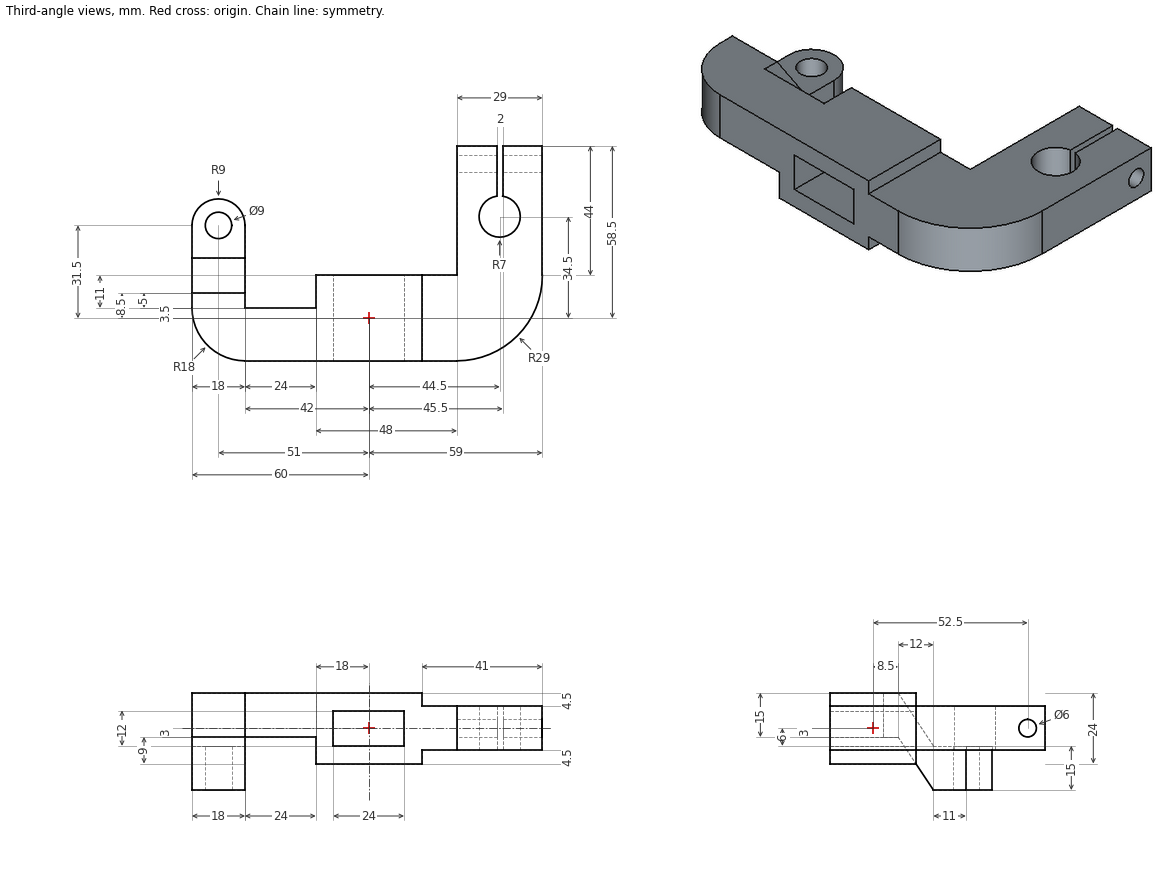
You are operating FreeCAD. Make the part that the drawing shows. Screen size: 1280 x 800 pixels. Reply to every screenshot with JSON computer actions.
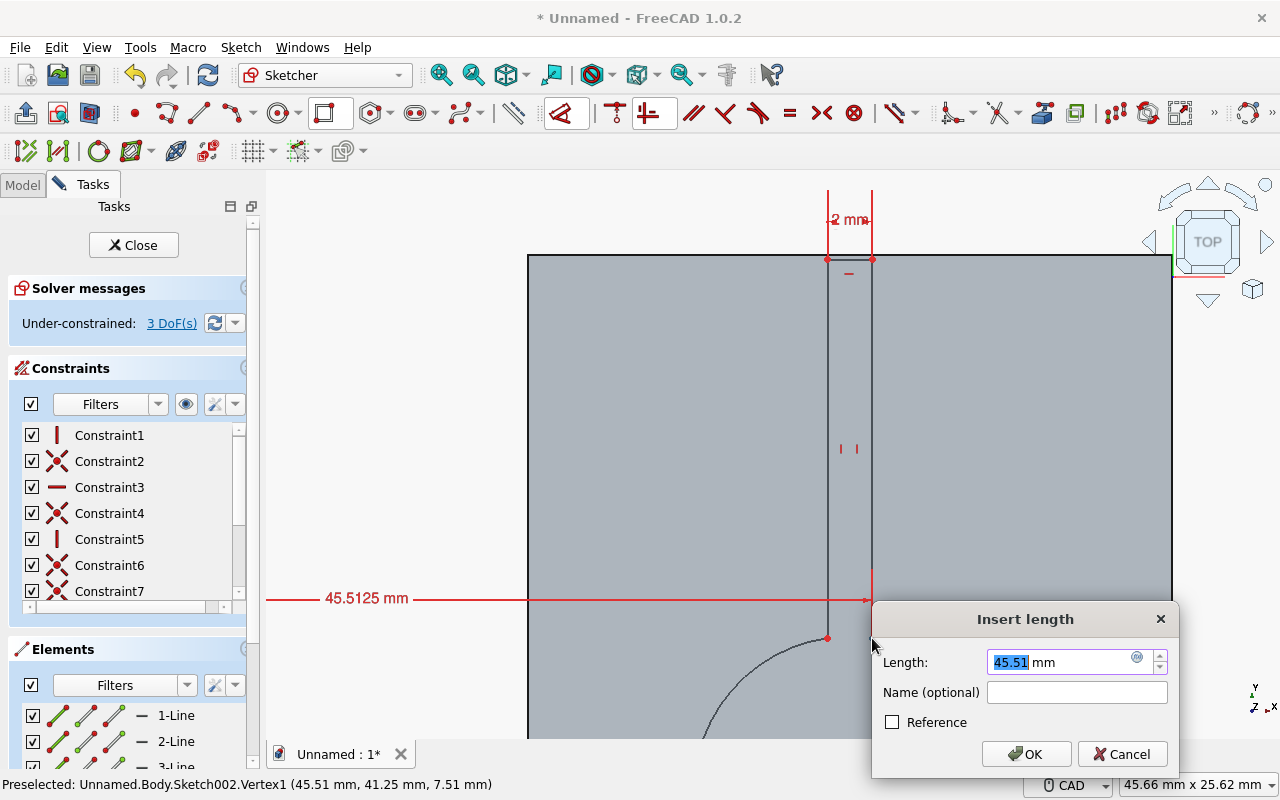
{"action": "type", "text": "45.5"}
{"action": "key", "text": "Return"}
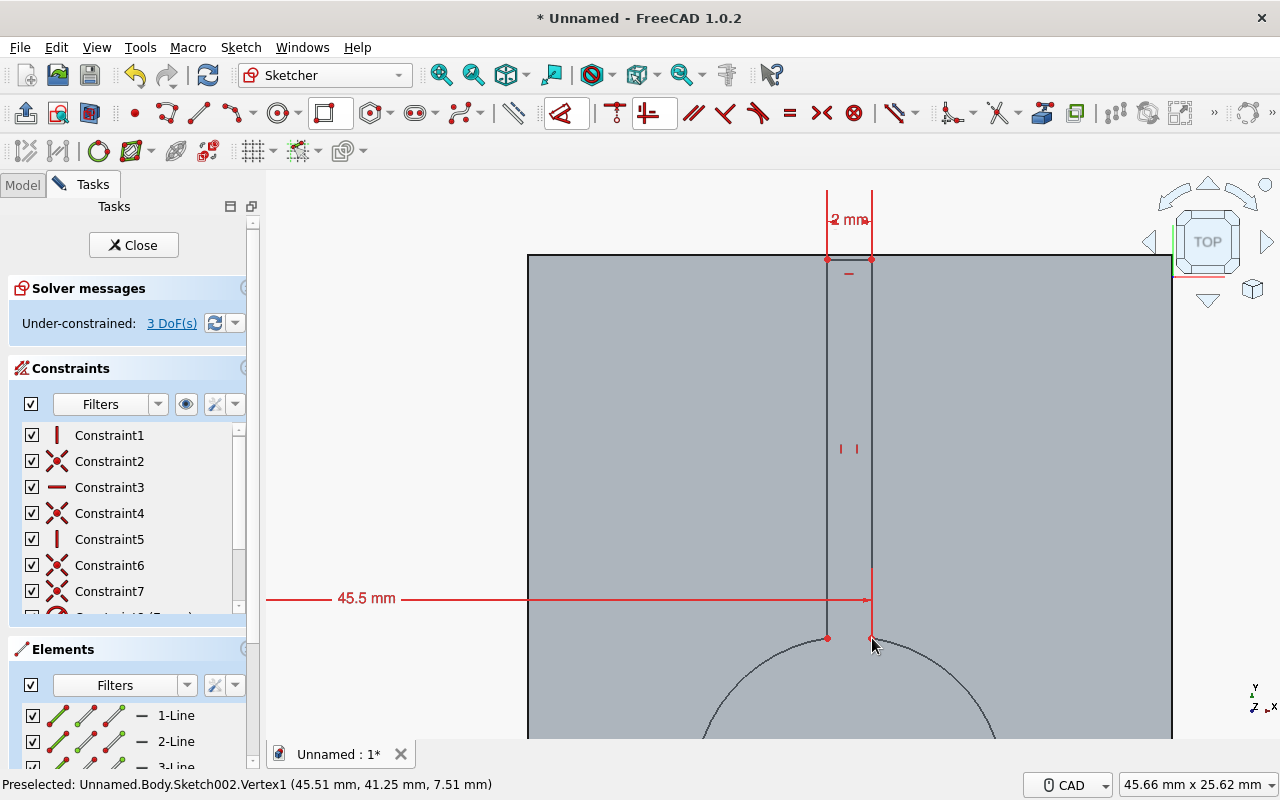
{"action": "left_click", "coordinate": [872, 260]}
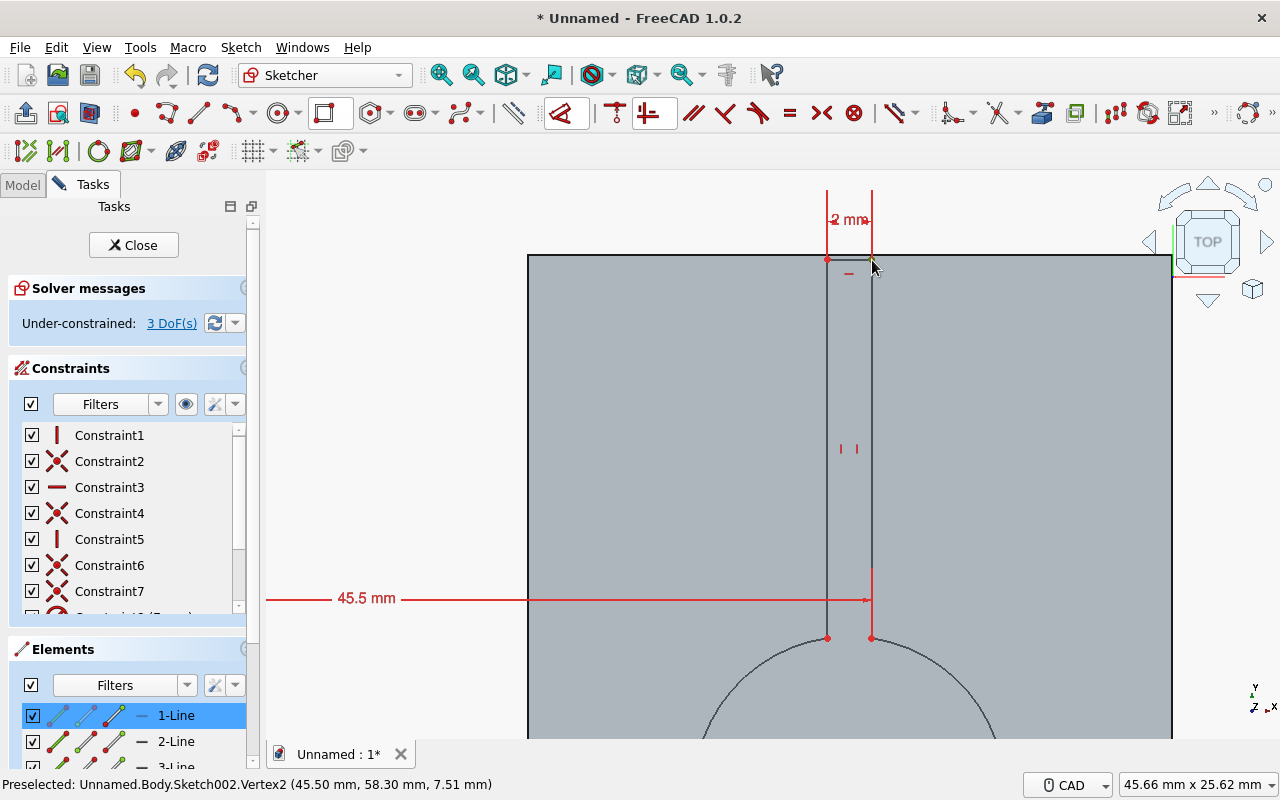
{"action": "left_click", "coordinate": [584, 114]}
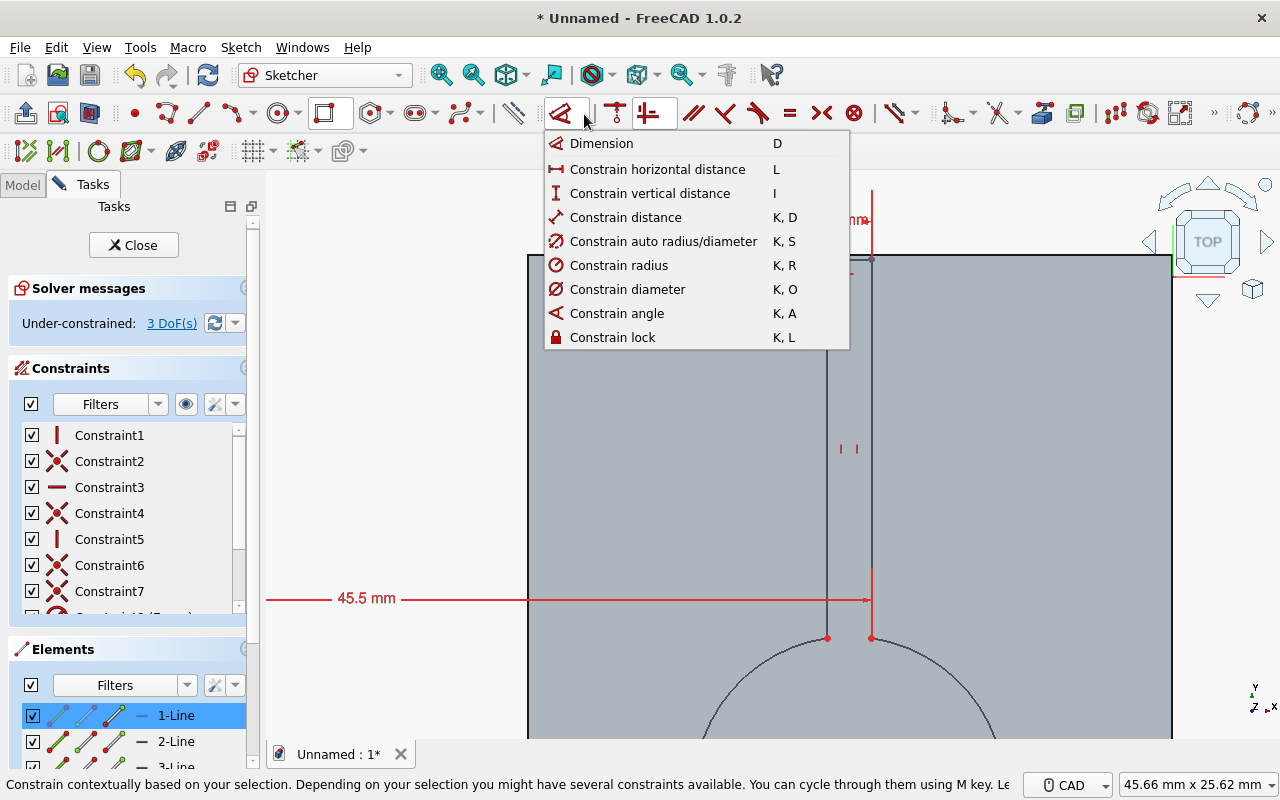
{"action": "left_click", "coordinate": [697, 193]}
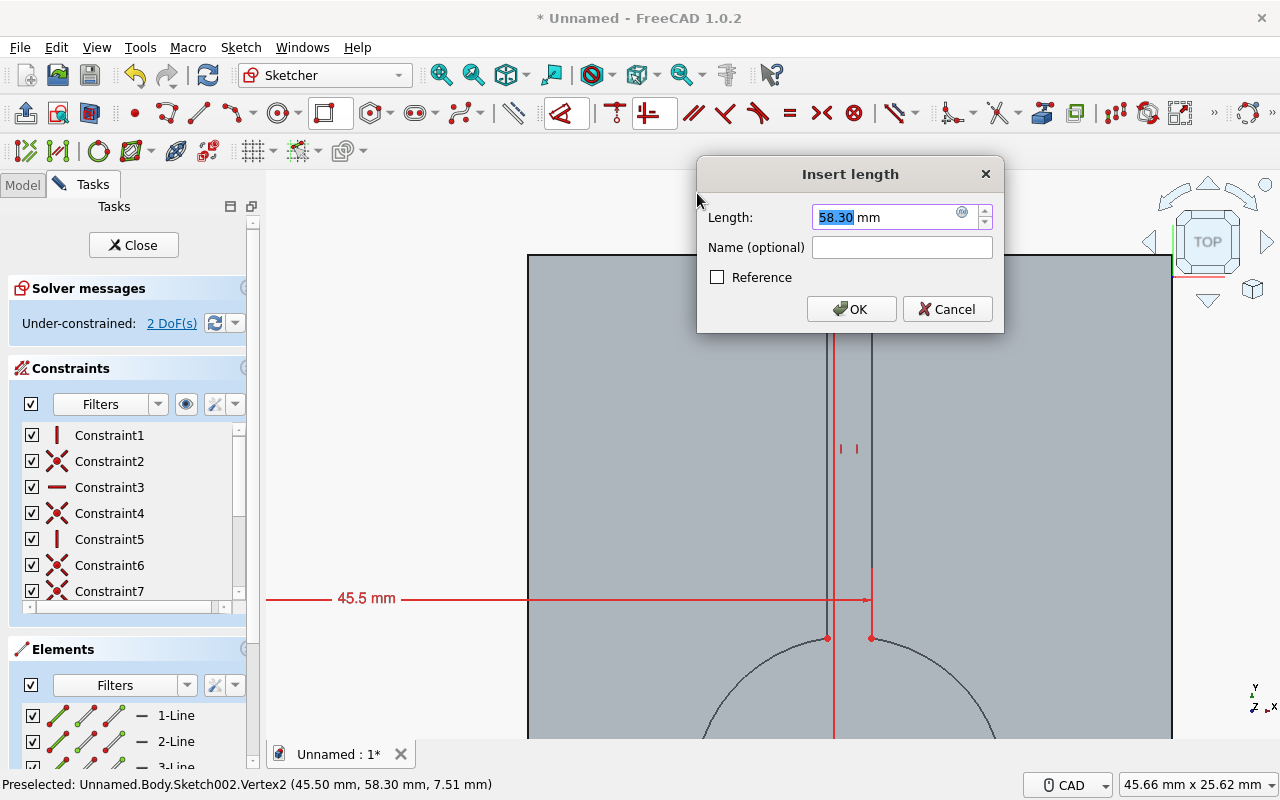
{"action": "type", "text": "58.5"}
{"action": "key", "text": "Return"}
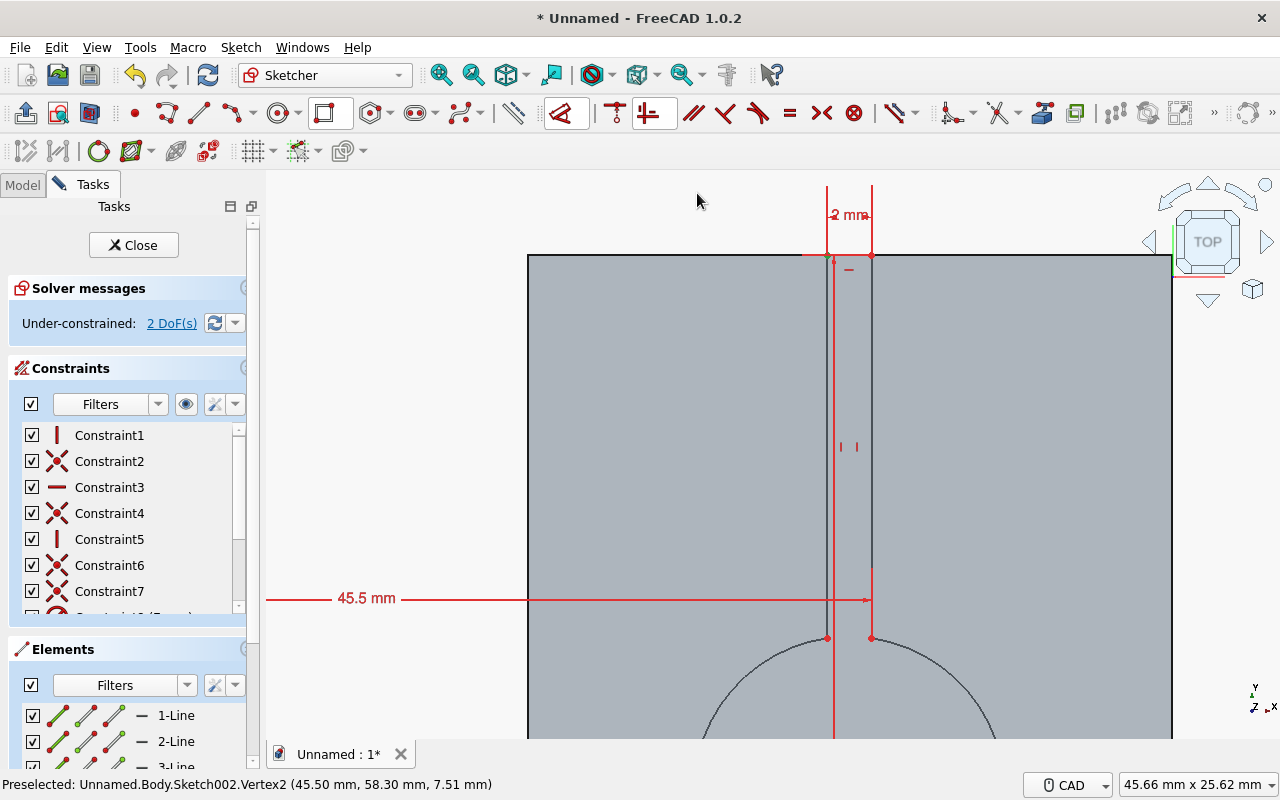
{"action": "scroll", "coordinate": [850, 260], "scroll_direction": "down", "scroll_amount": 6}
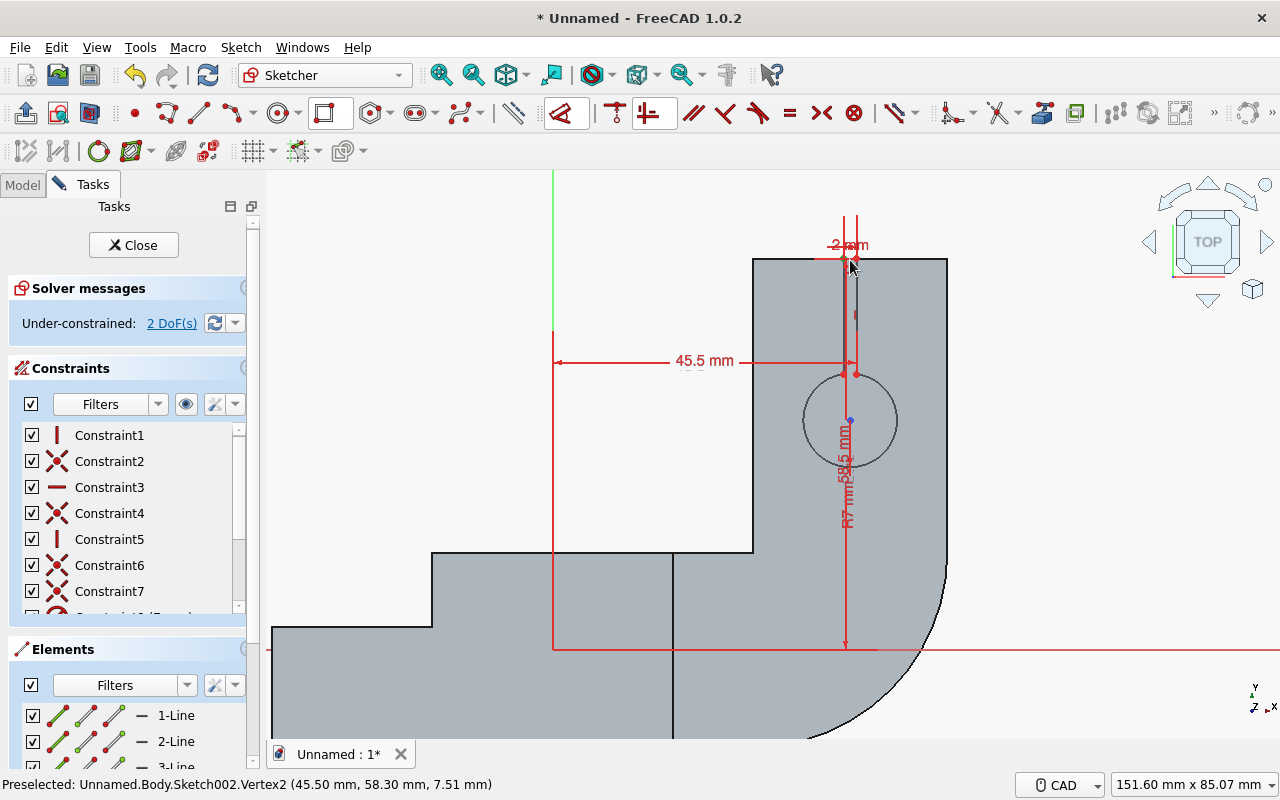
{"action": "left_click", "coordinate": [850, 420]}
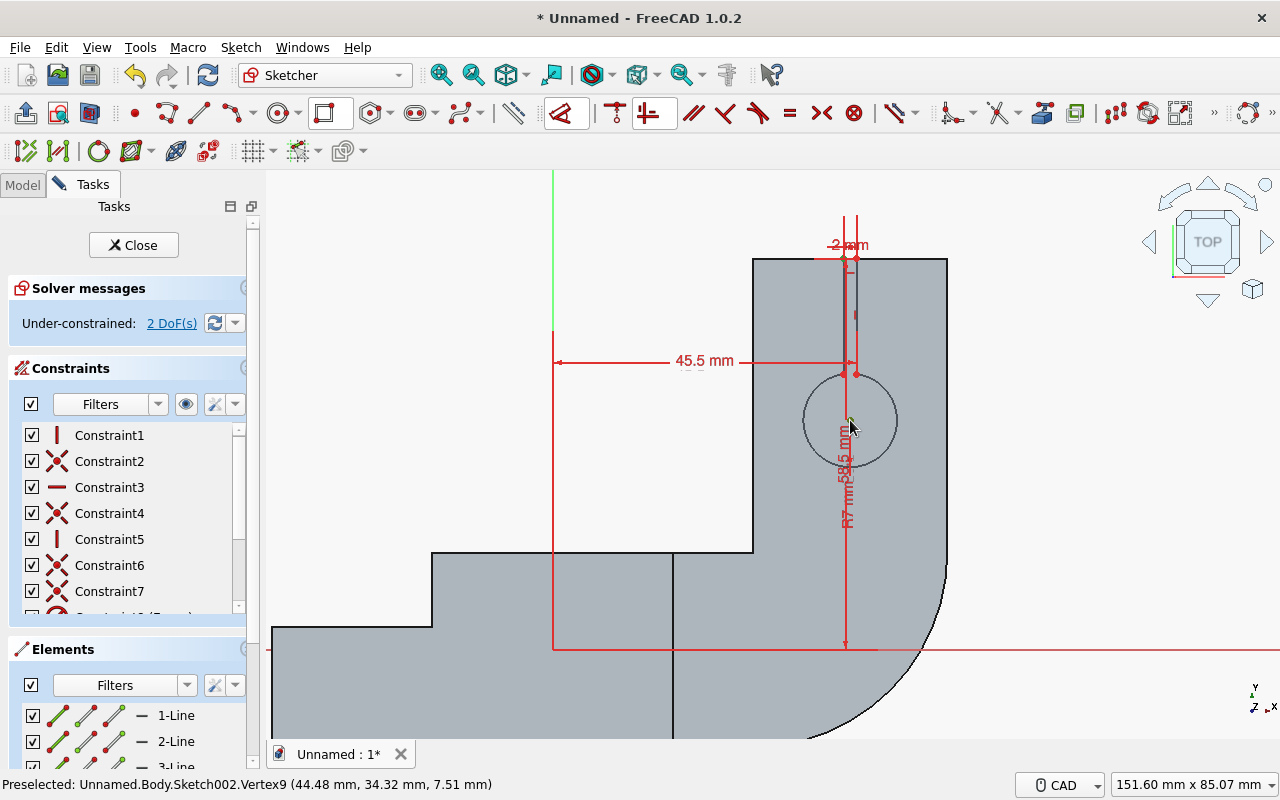
{"action": "key", "text": "l"}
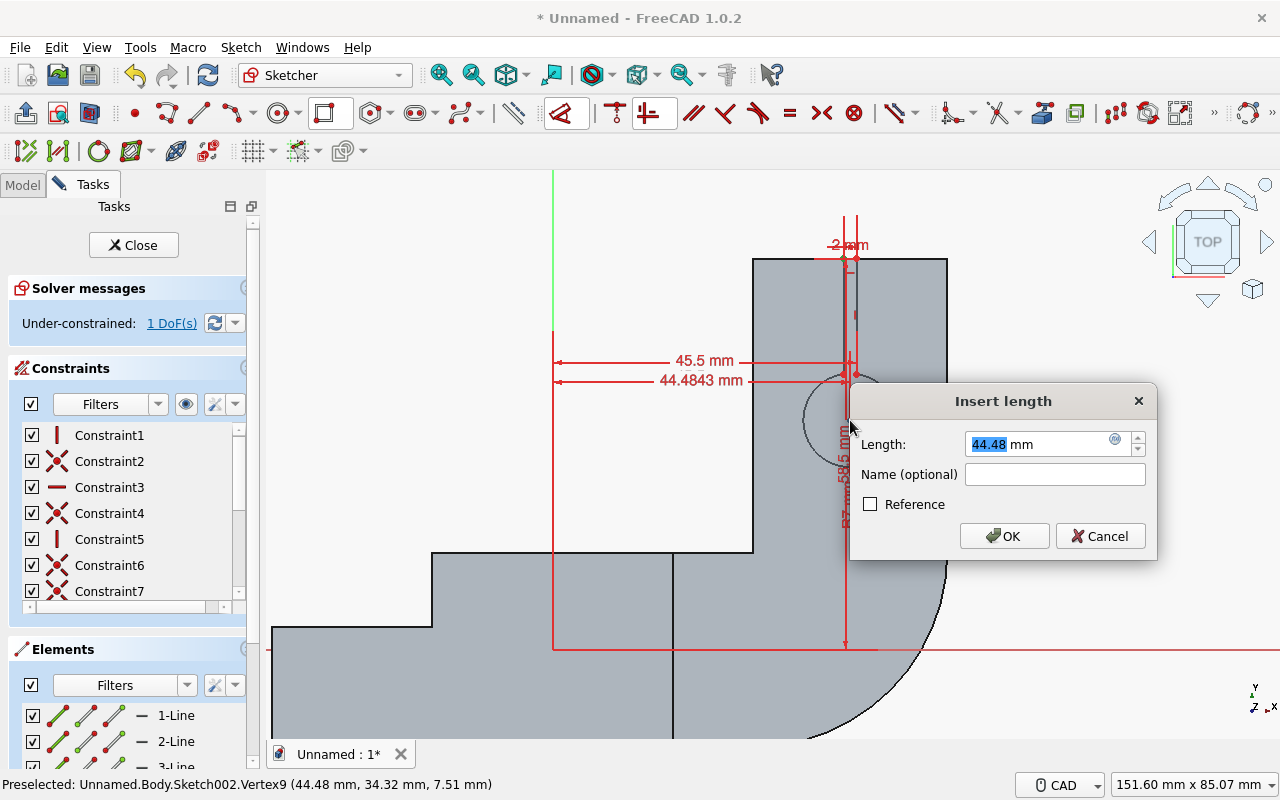
{"action": "type", "text": "44.5"}
{"action": "key", "text": "Return"}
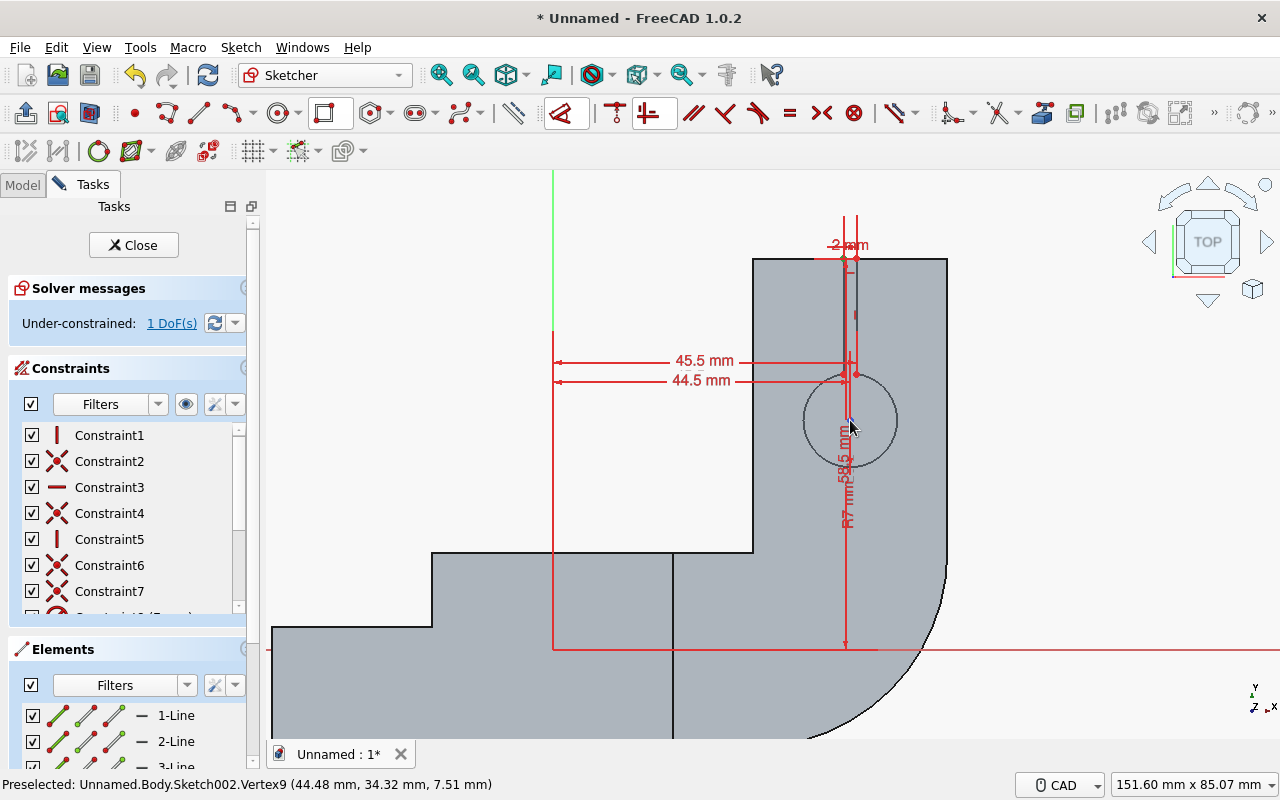
{"action": "left_click", "coordinate": [850, 420]}